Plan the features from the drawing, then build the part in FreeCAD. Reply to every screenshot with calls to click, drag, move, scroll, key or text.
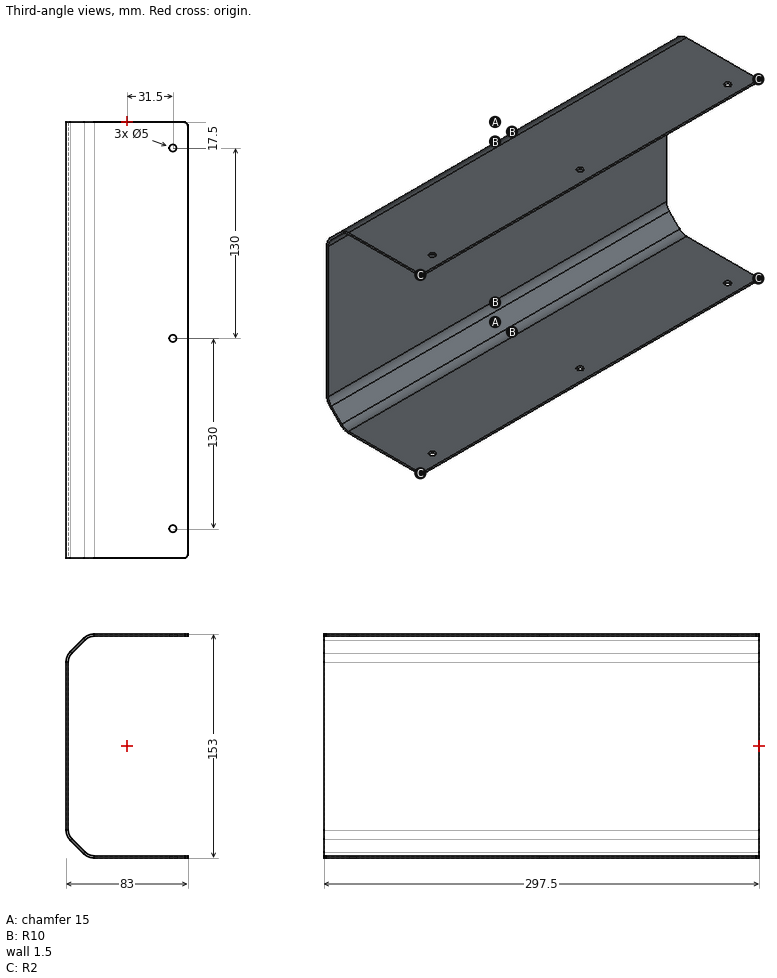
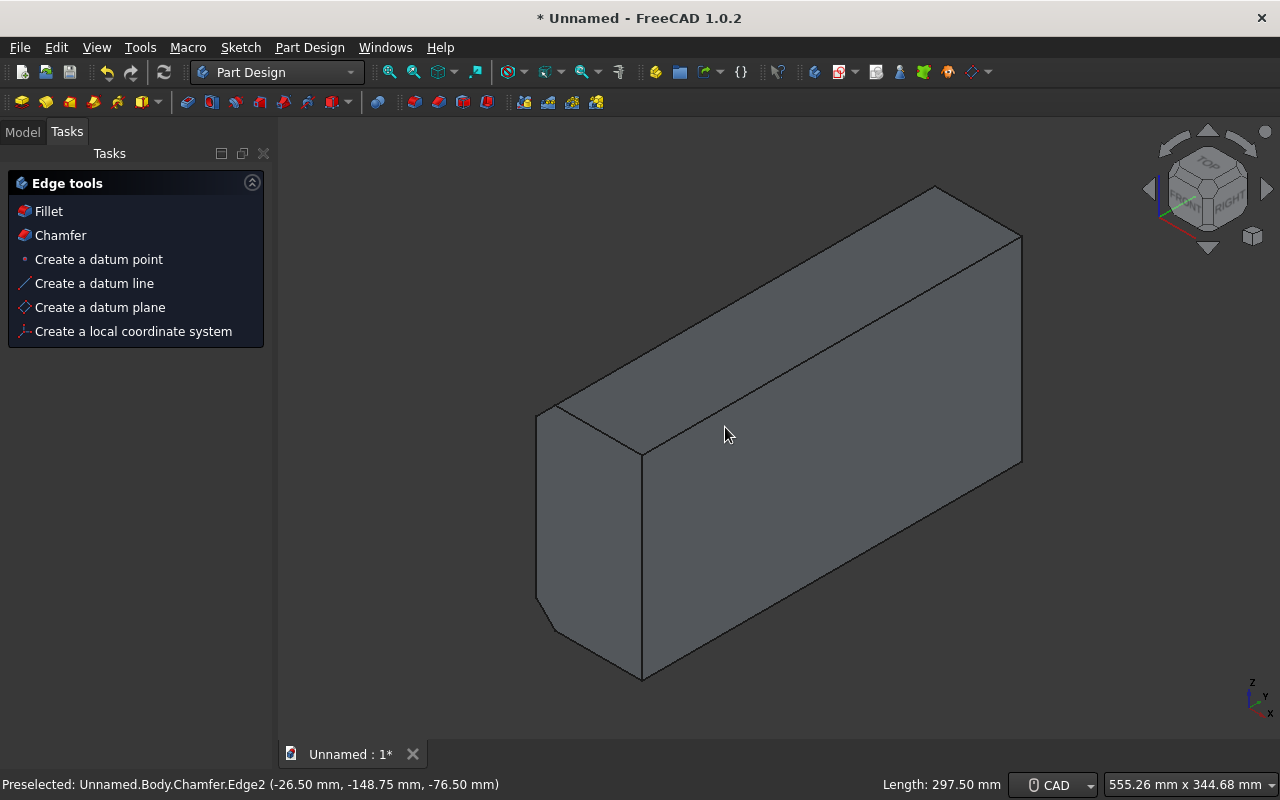
key(2)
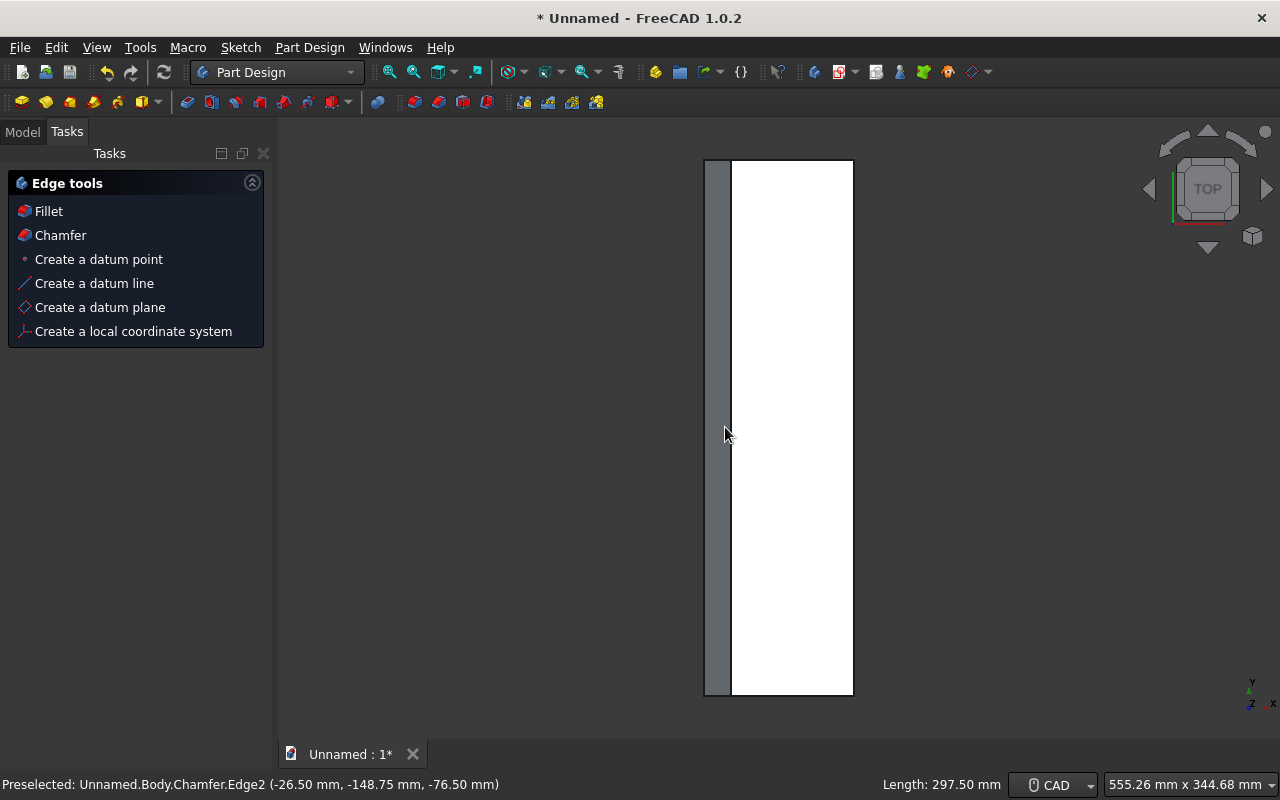
click(731, 427, ctrl)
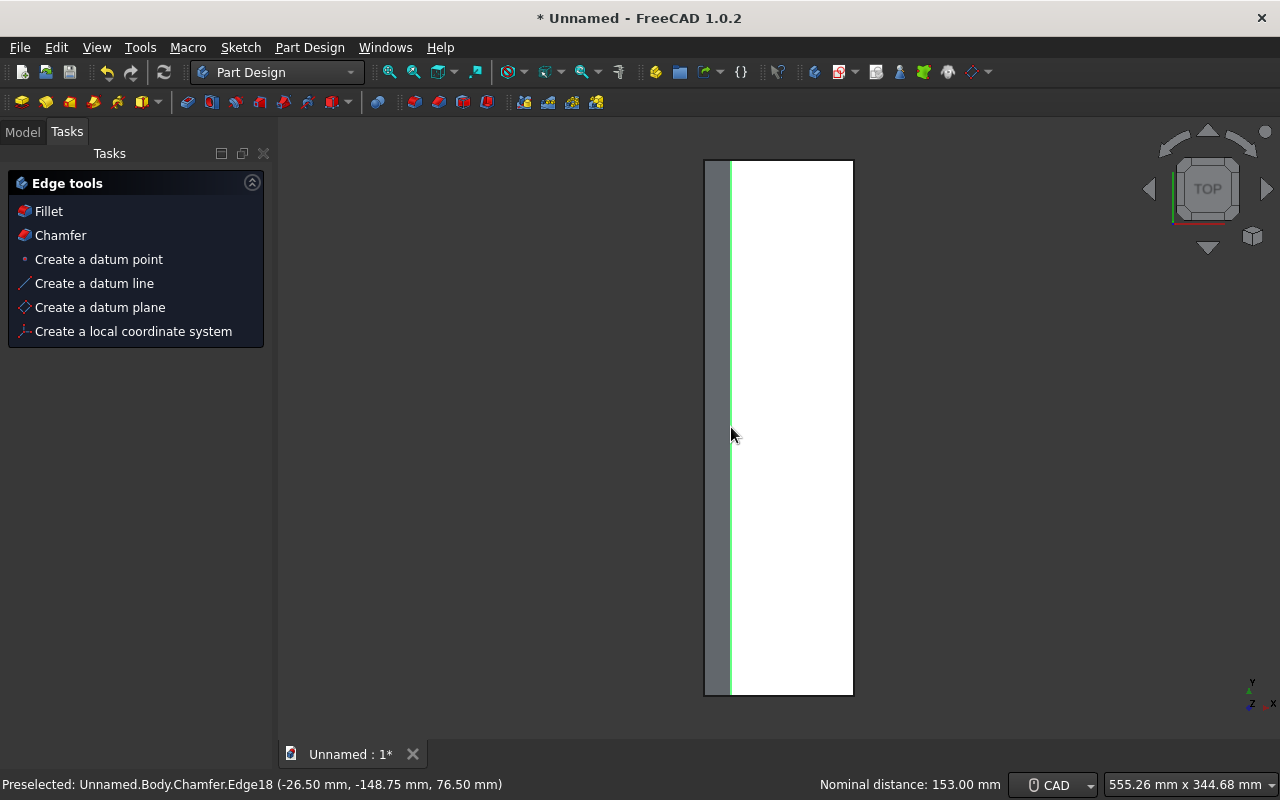
key(1)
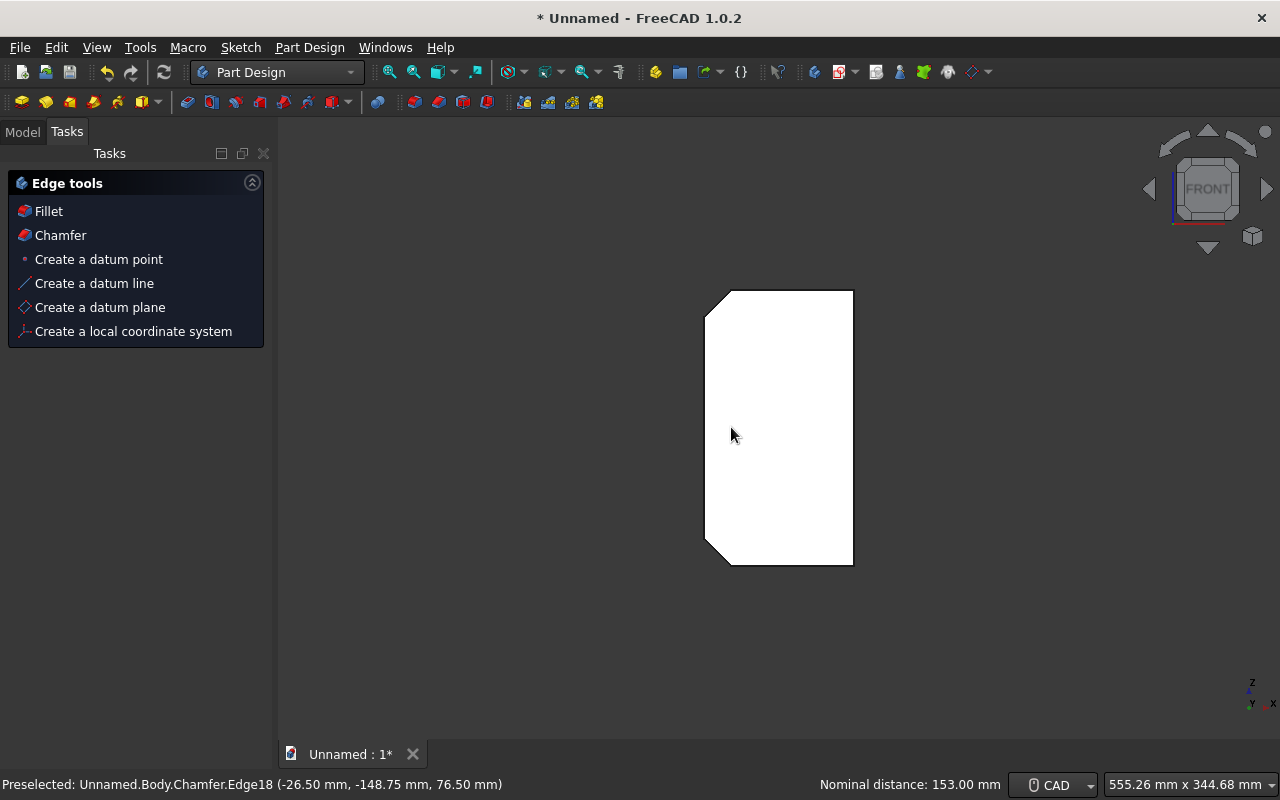
key(v)
key(f)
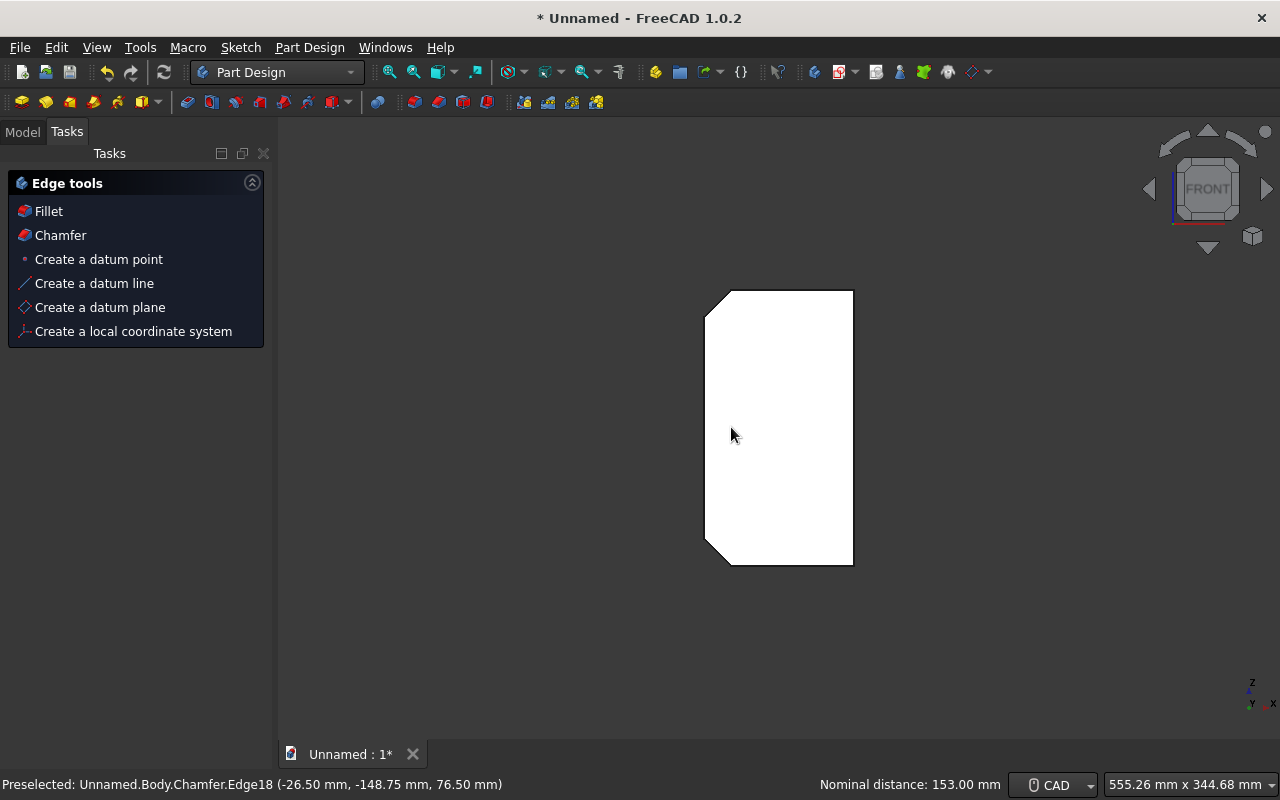
key(3)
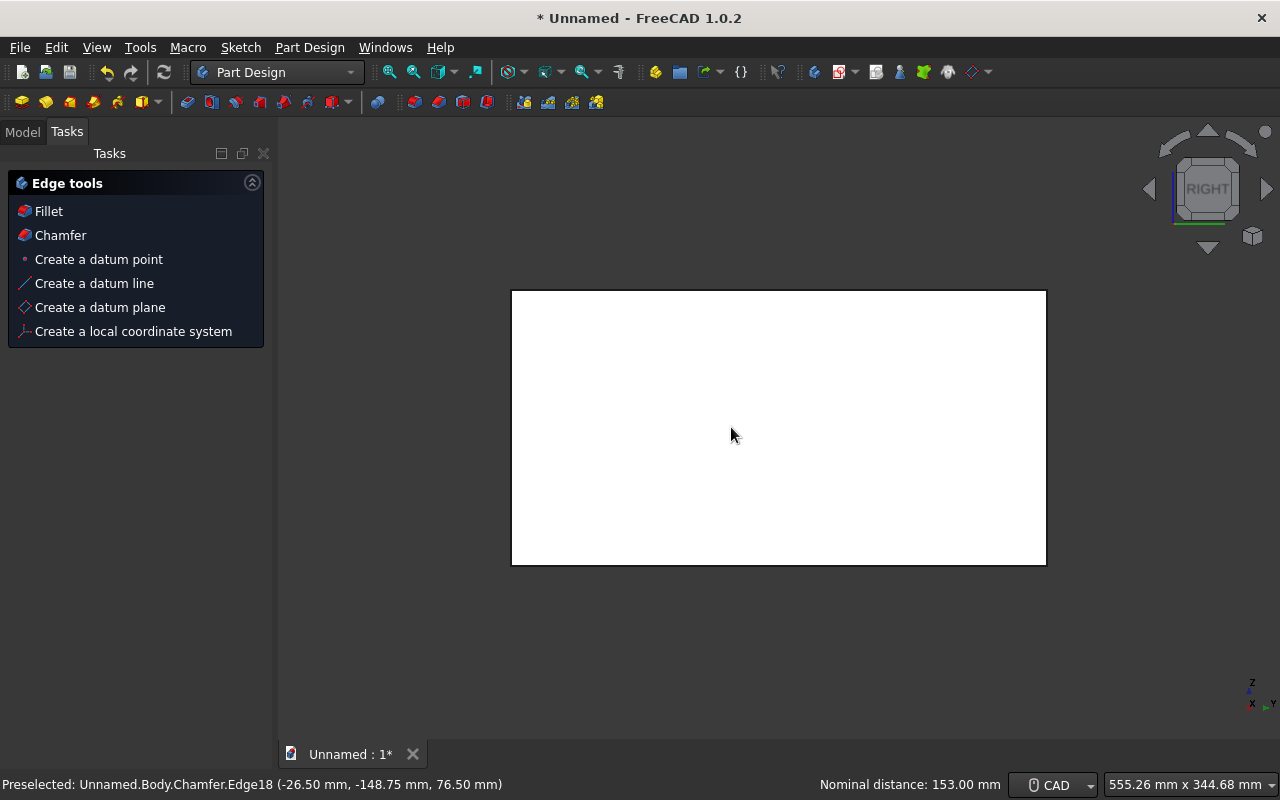
key(5)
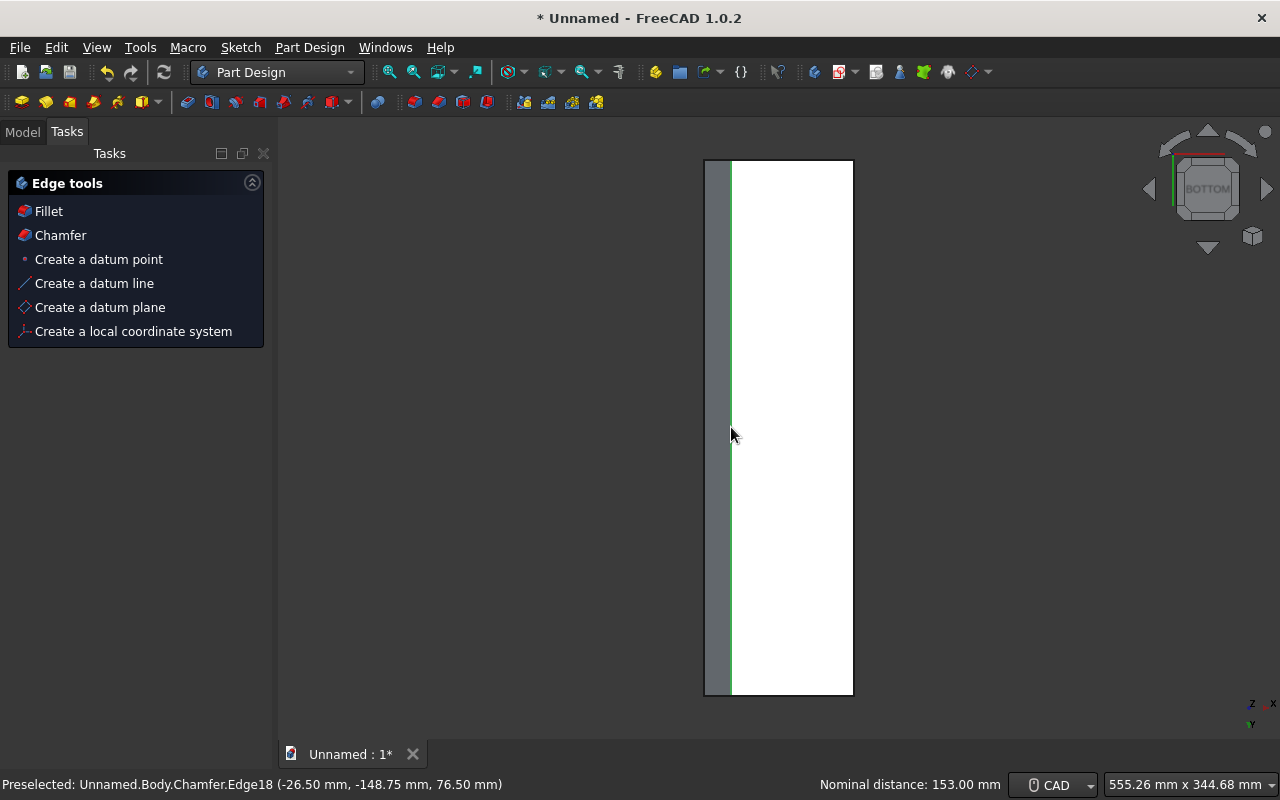
key(4)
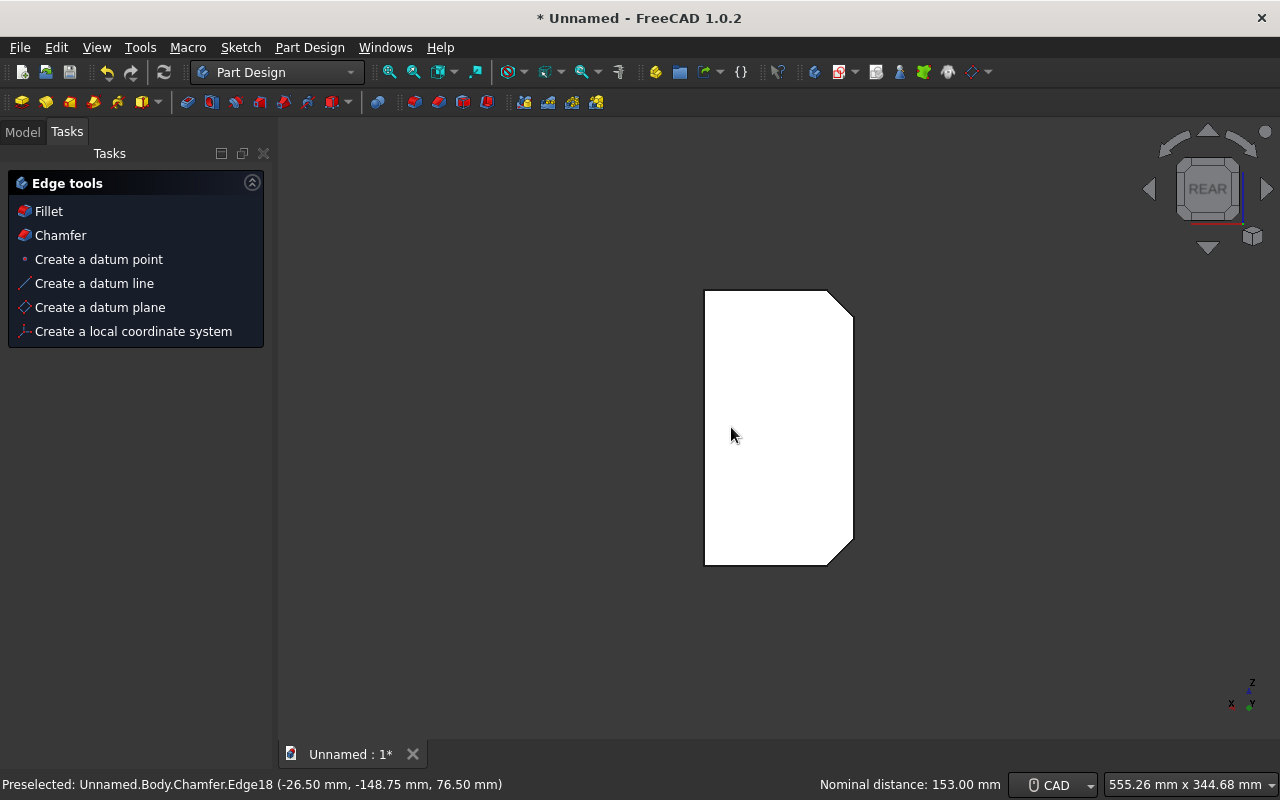
key(v)
key(f)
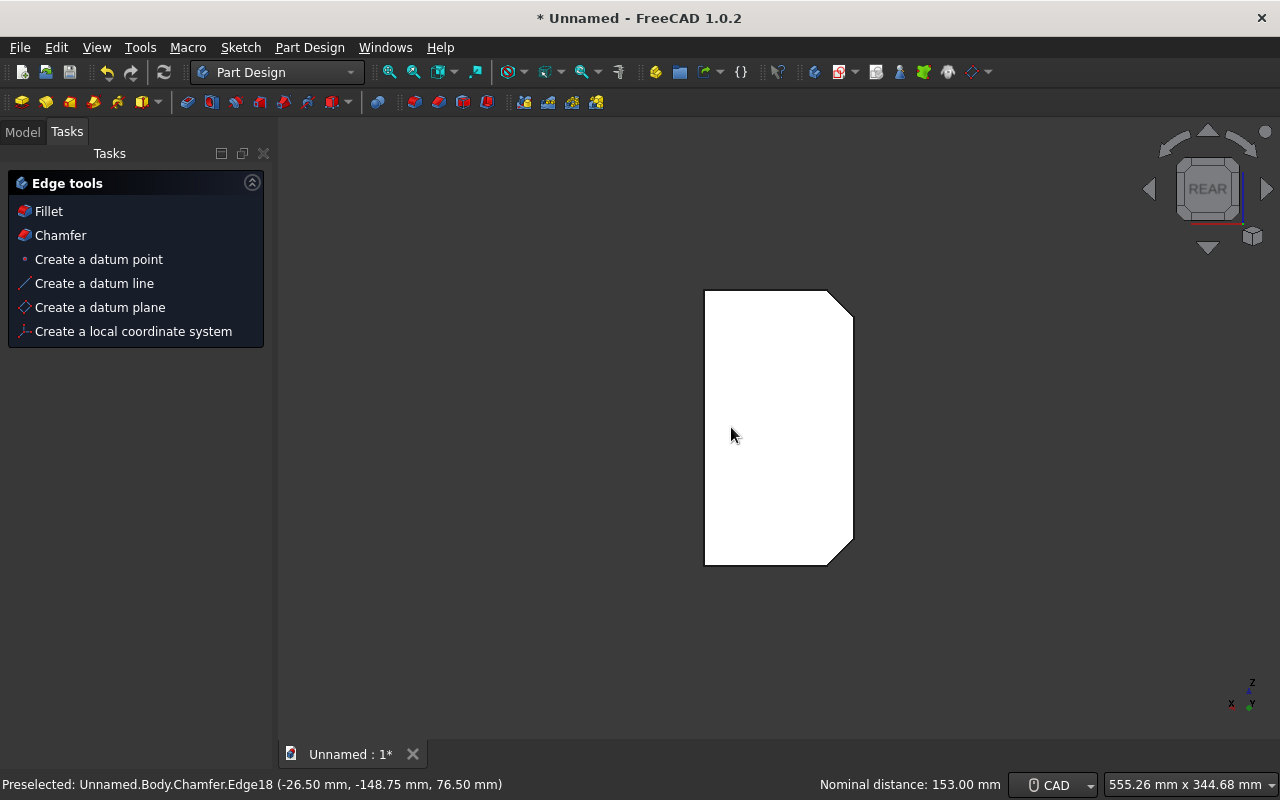
key(6)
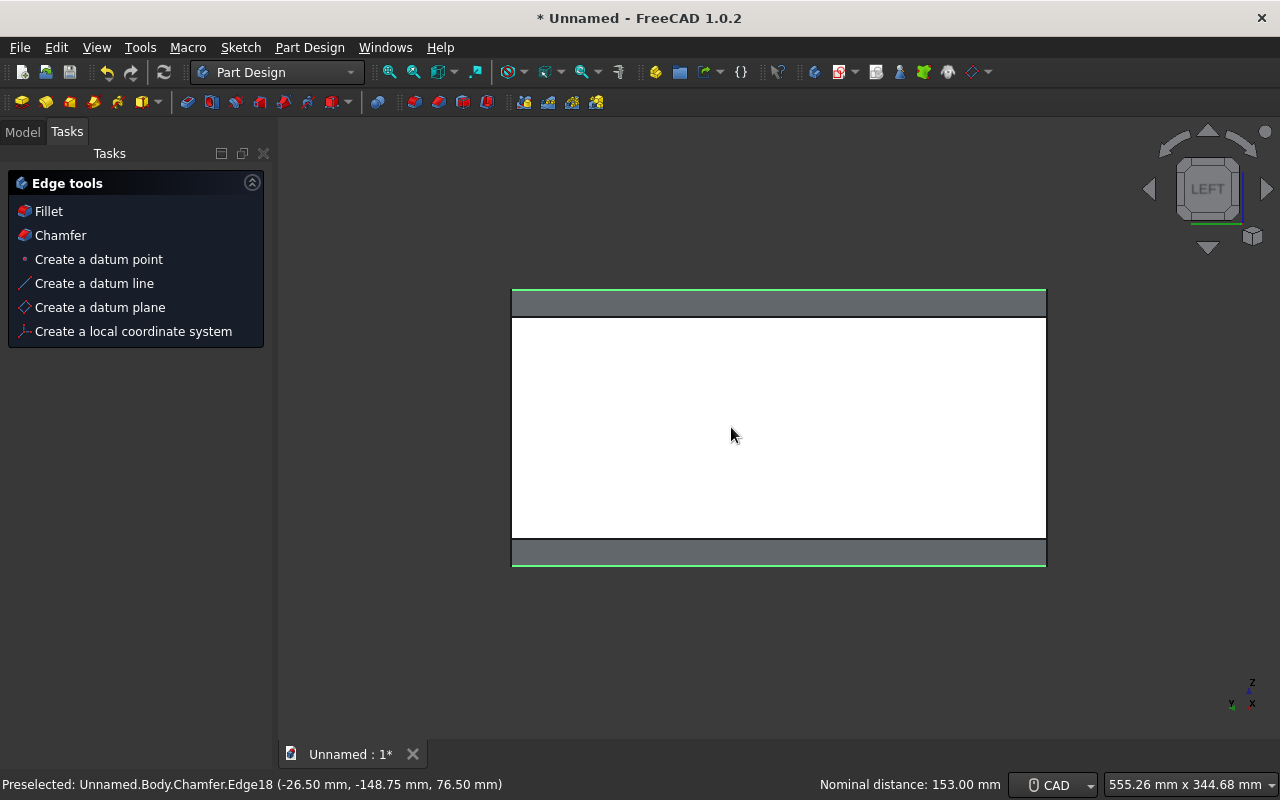
click(779, 316, ctrl)